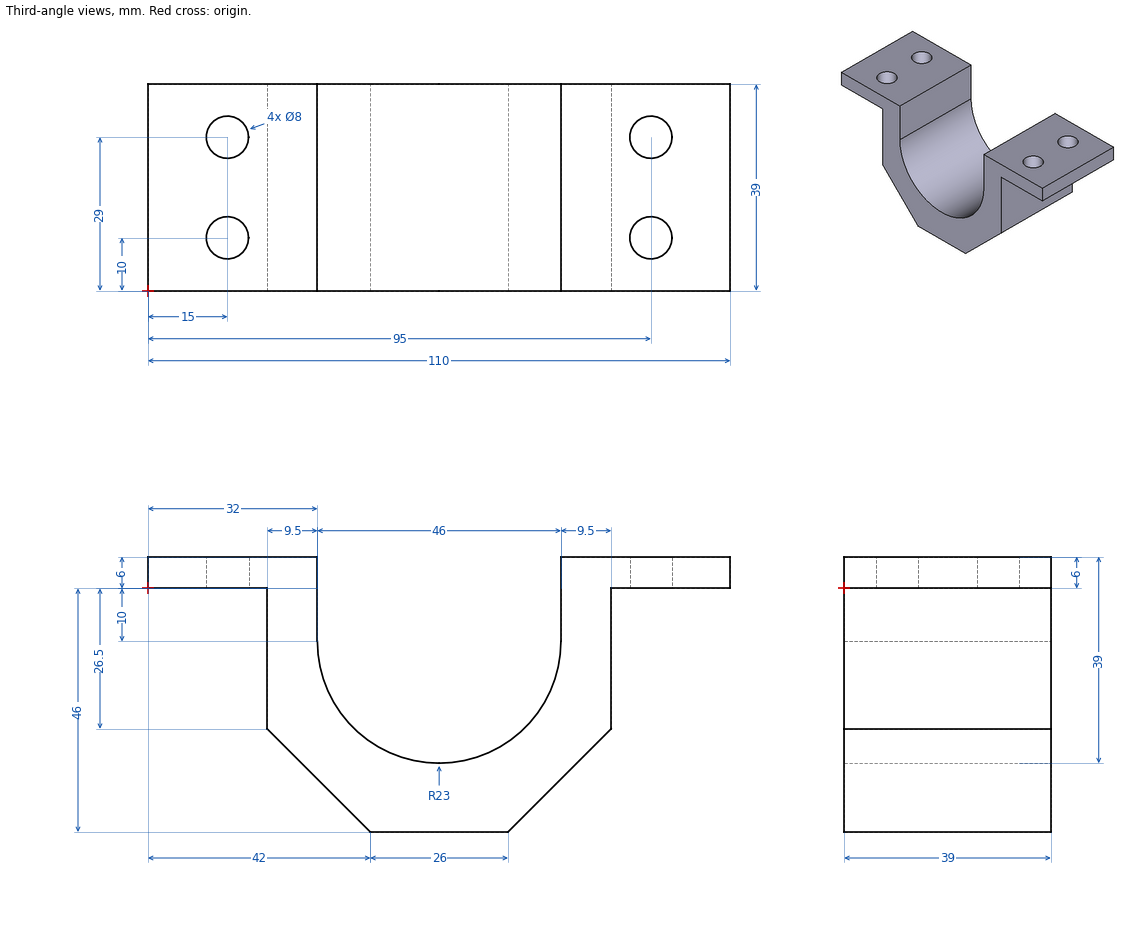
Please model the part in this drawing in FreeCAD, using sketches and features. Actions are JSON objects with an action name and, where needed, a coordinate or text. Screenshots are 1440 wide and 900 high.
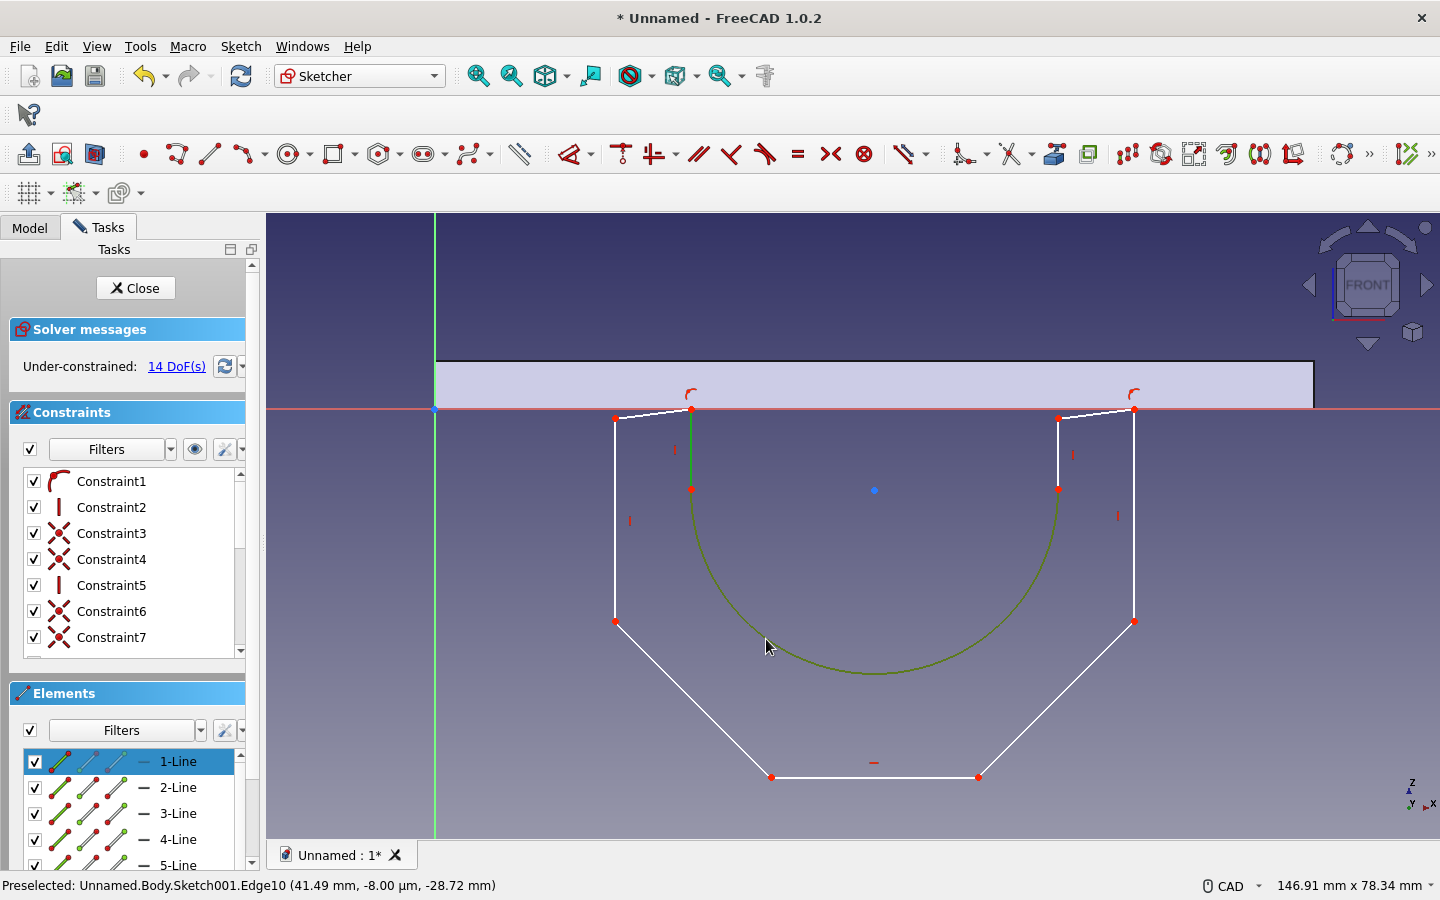
{"action": "left_click", "coordinate": [765, 154]}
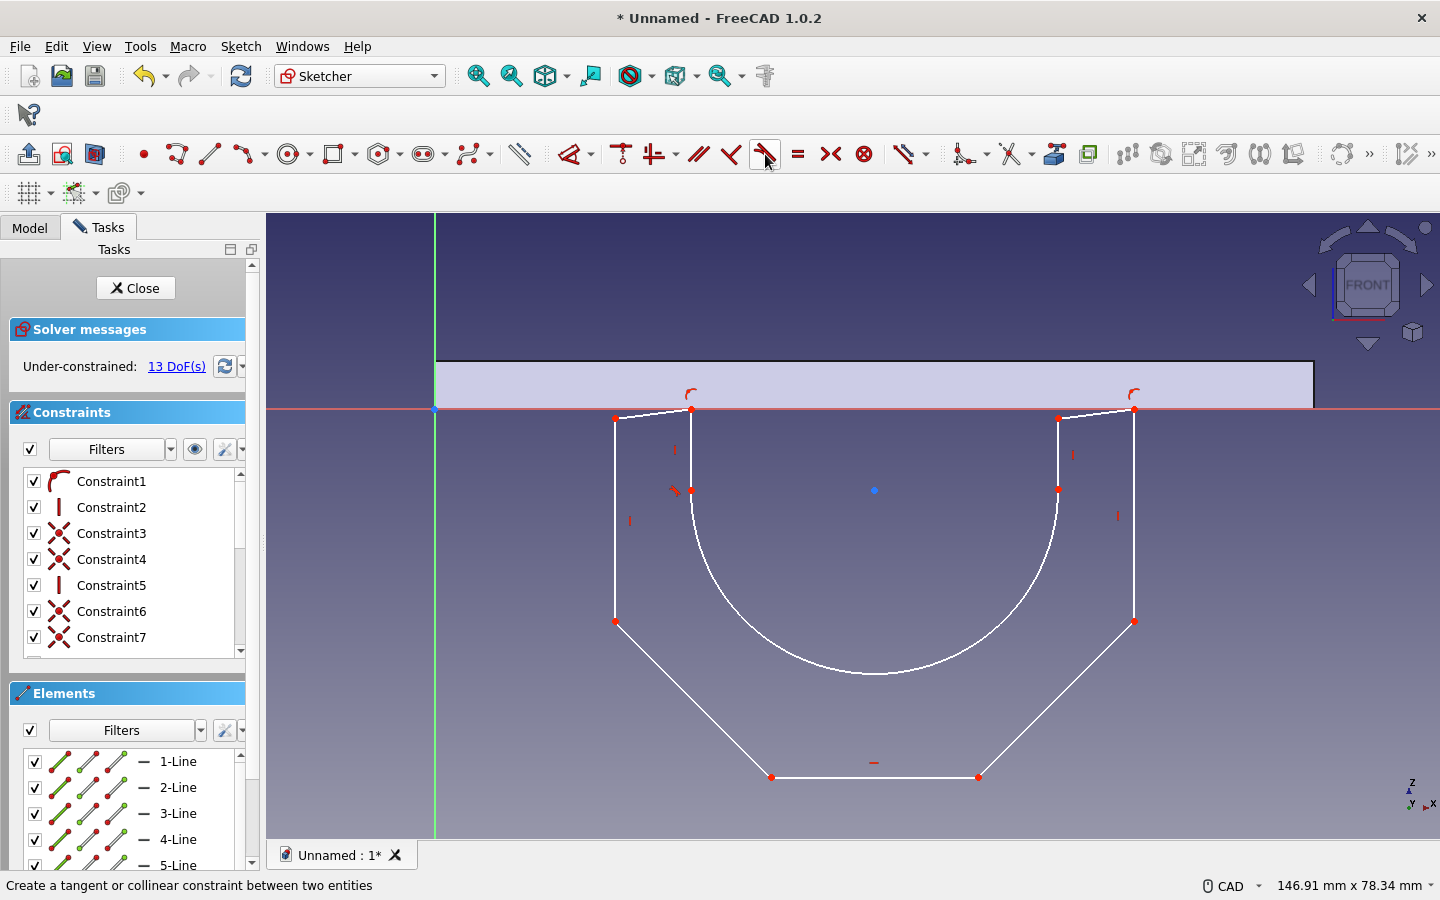
{"action": "left_click", "coordinate": [1058, 440]}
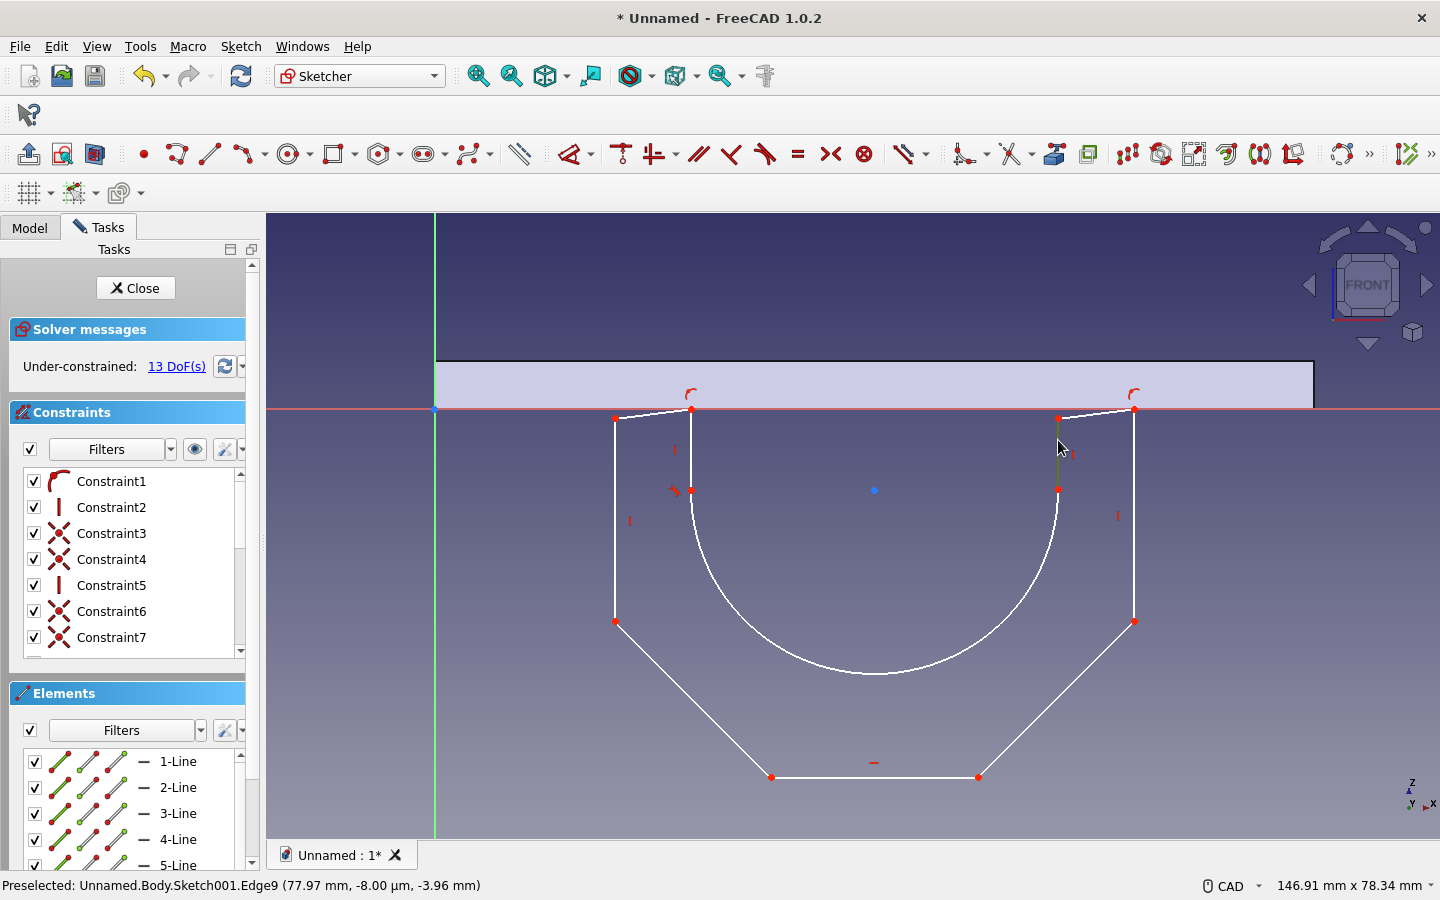
{"action": "left_click", "coordinate": [767, 639]}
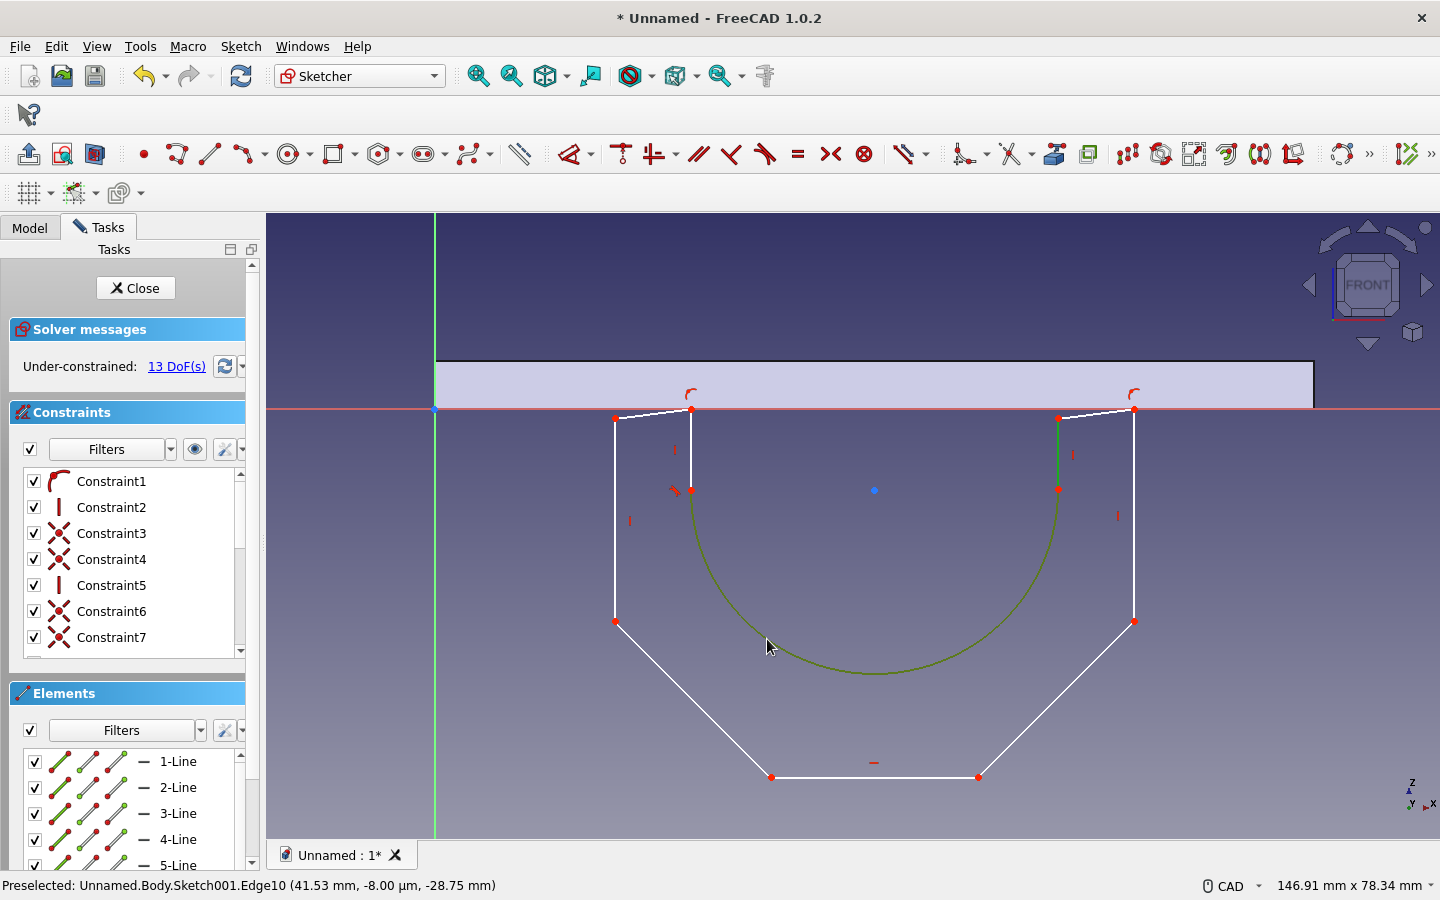
{"action": "left_click", "coordinate": [765, 154]}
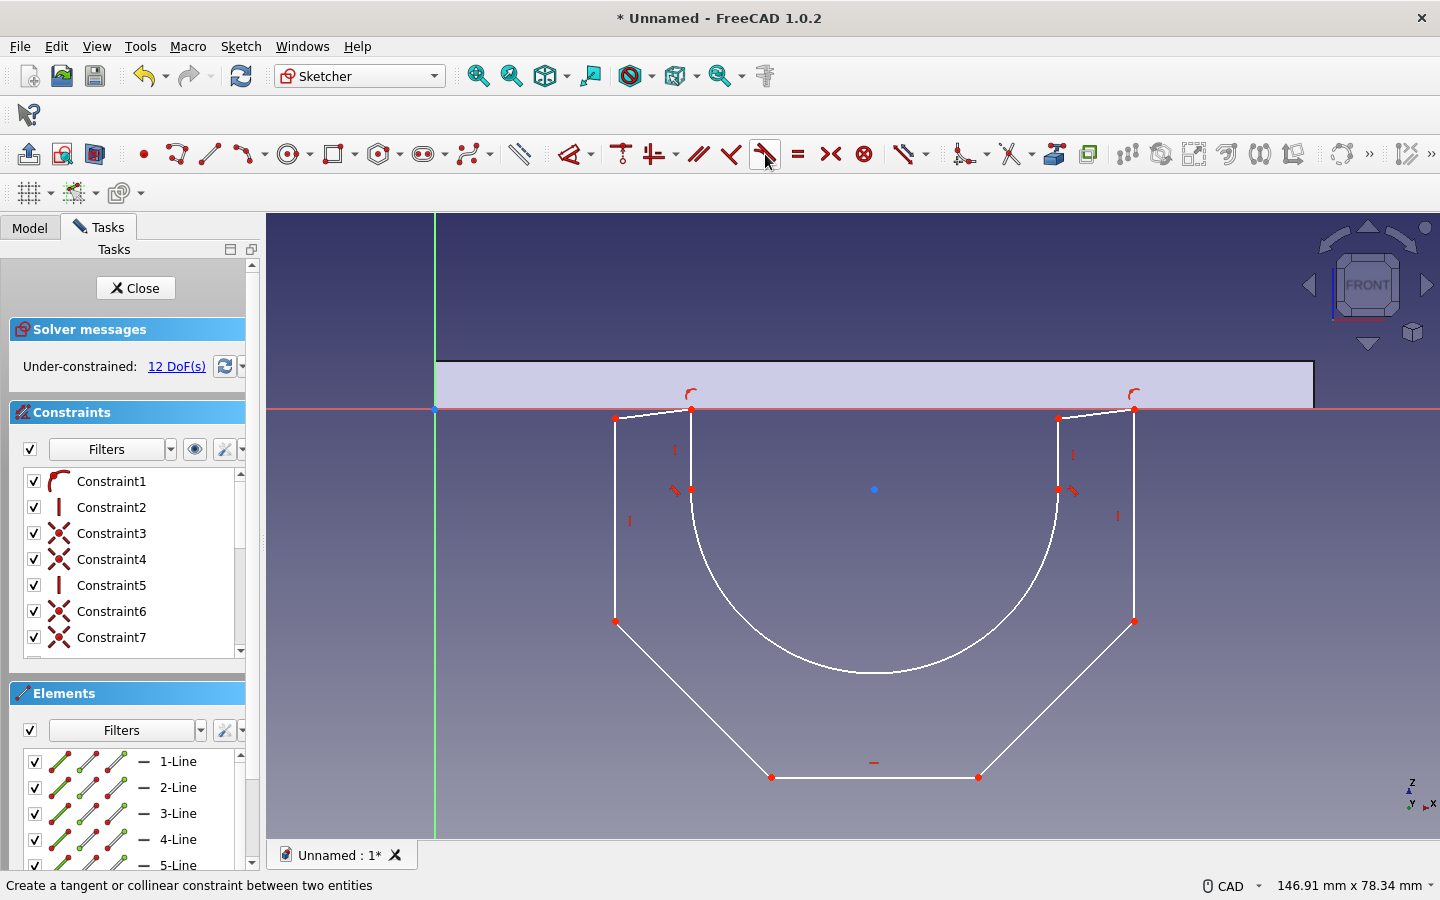
{"action": "left_click", "coordinate": [668, 412]}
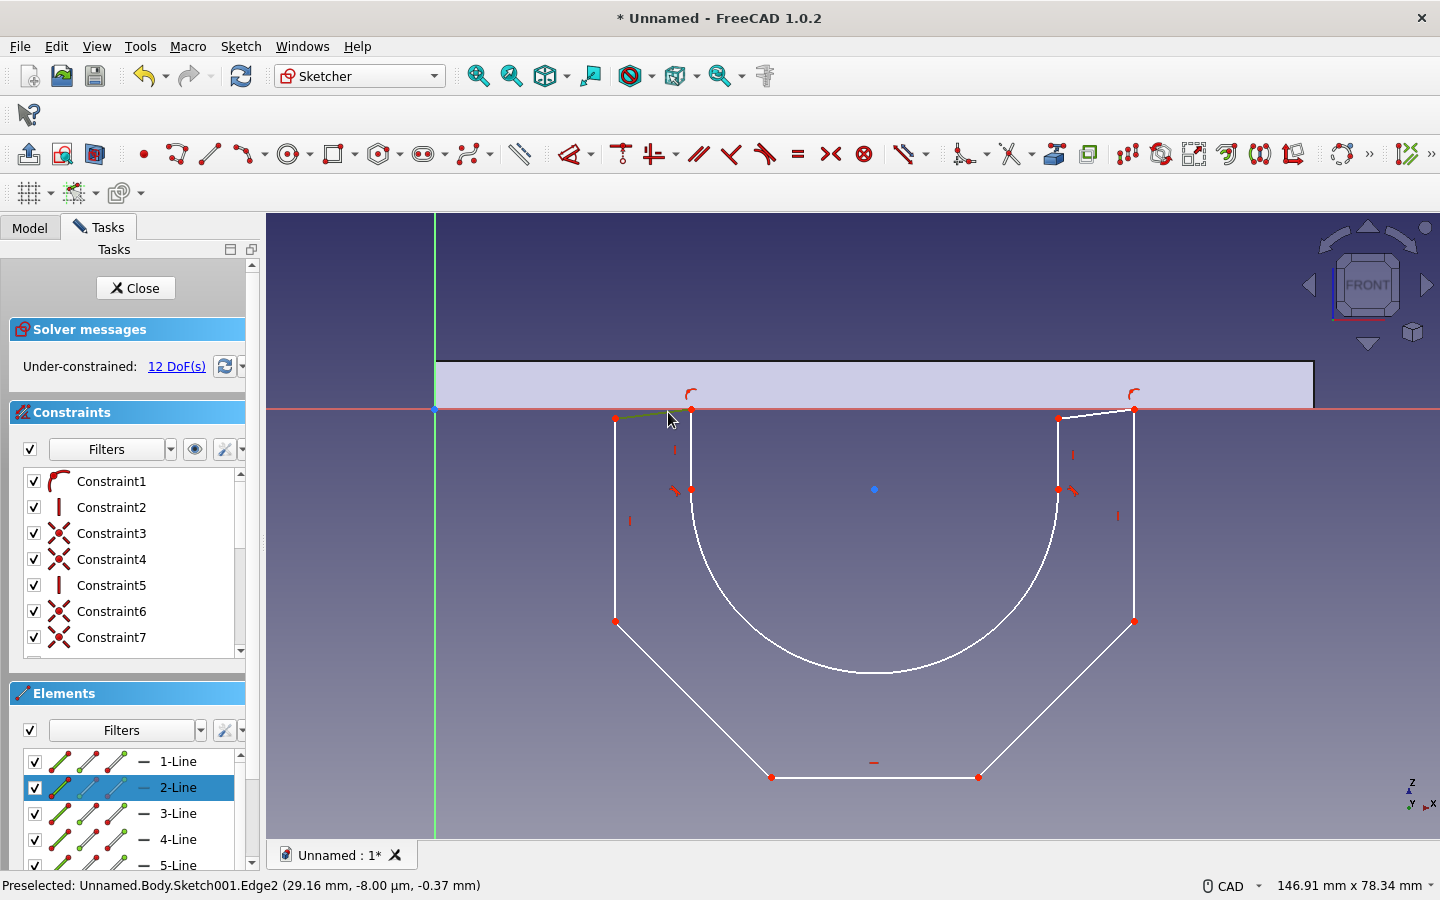
{"action": "key", "text": "h"}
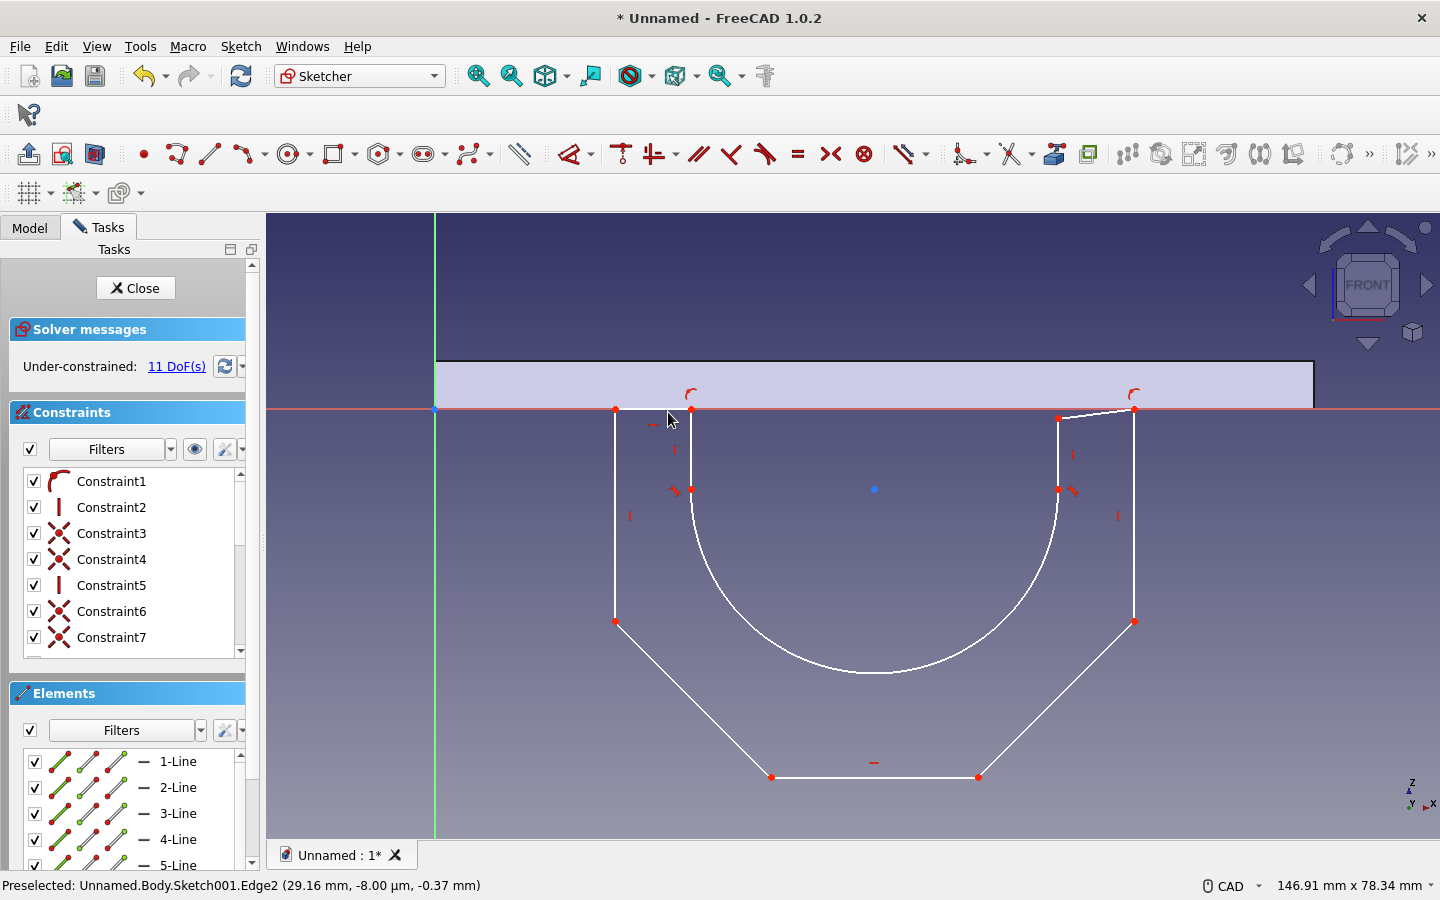
{"action": "left_click", "coordinate": [1111, 412]}